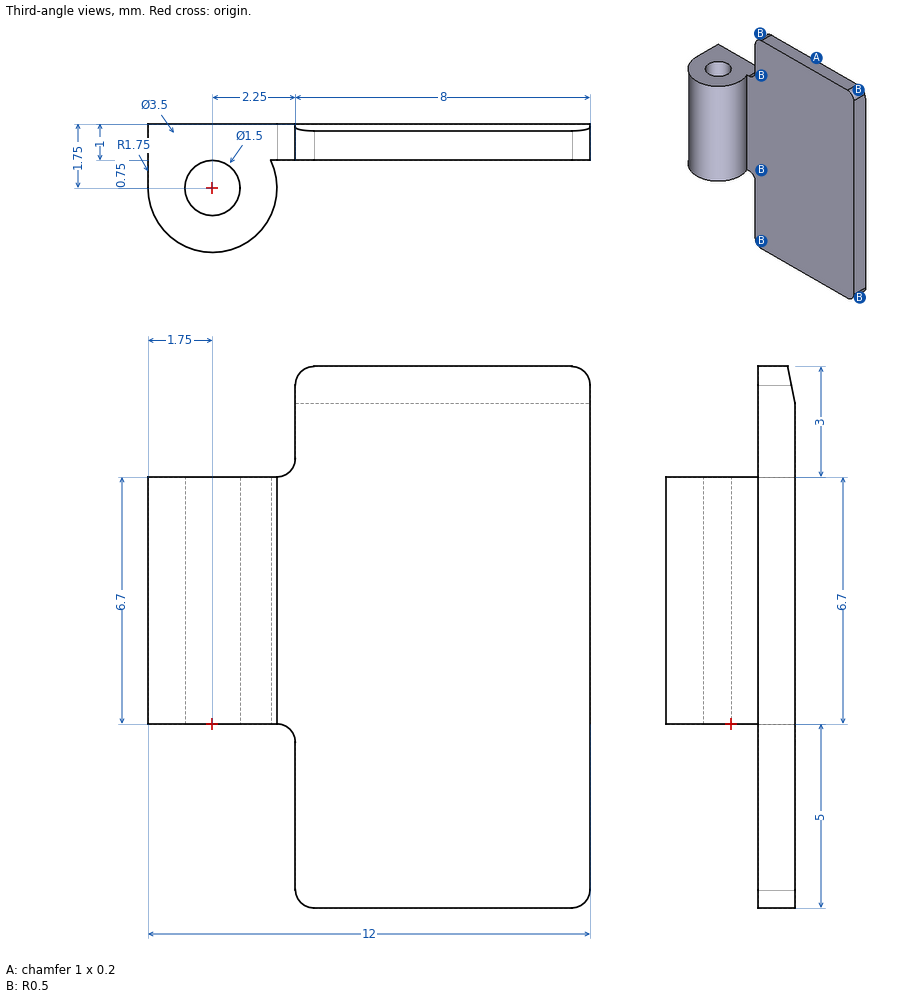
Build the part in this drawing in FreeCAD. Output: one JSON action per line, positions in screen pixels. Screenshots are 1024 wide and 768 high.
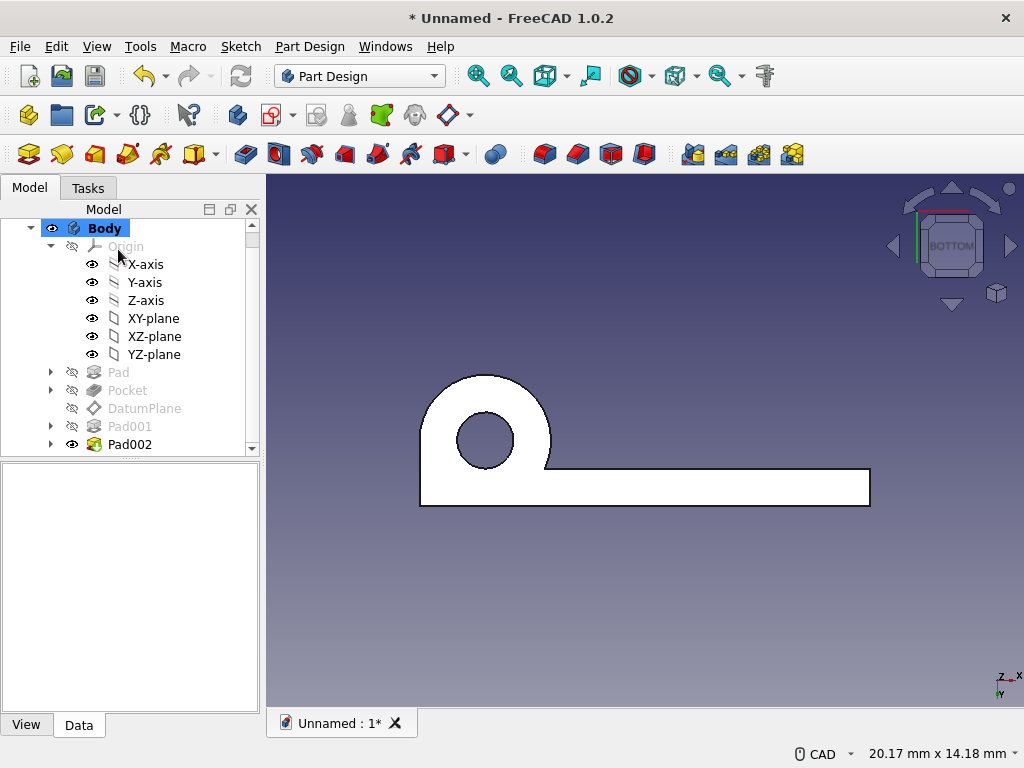
{"action": "key", "text": "0"}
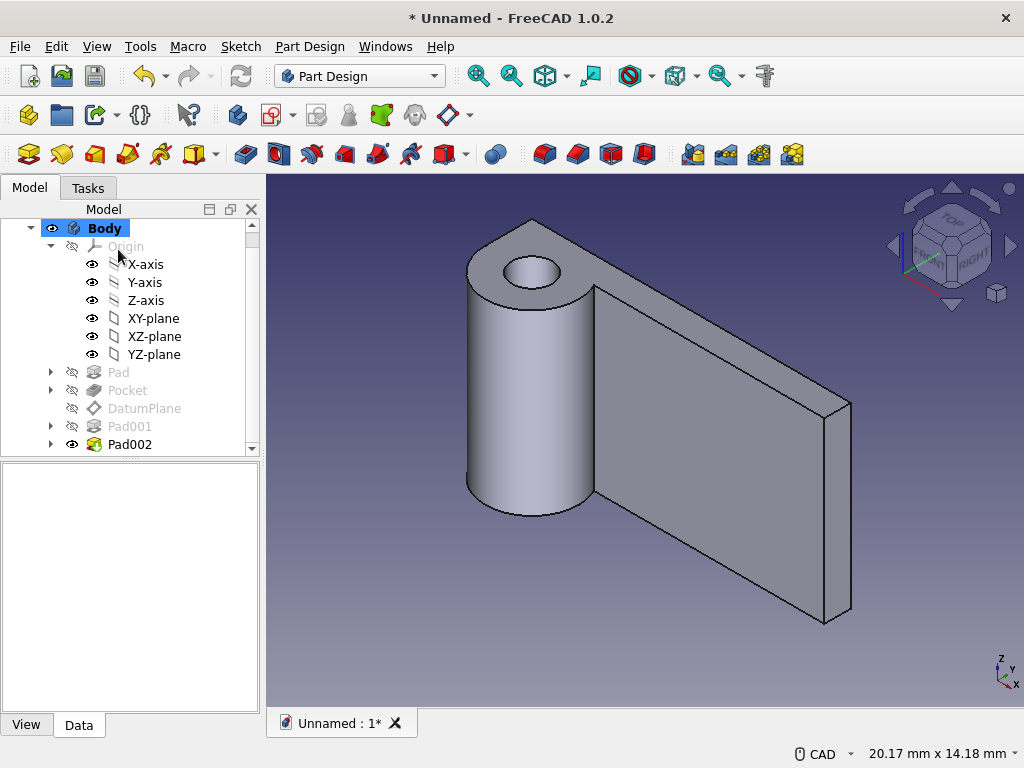
{"action": "left_click", "coordinate": [535, 242]}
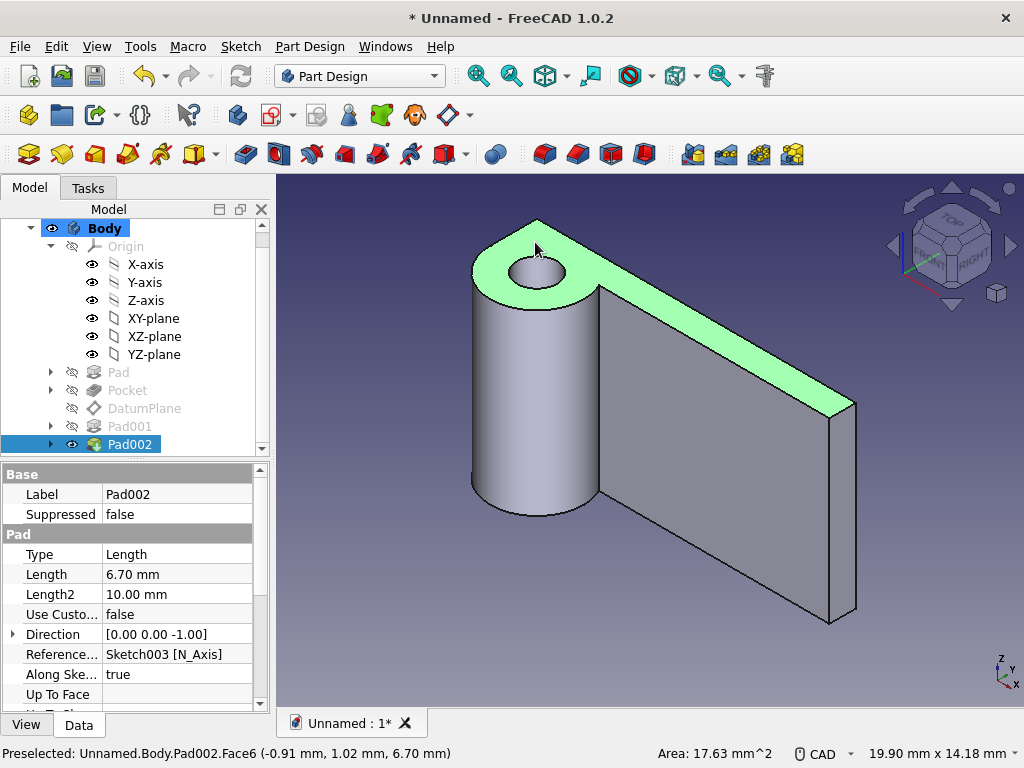
{"action": "left_click", "coordinate": [270, 116]}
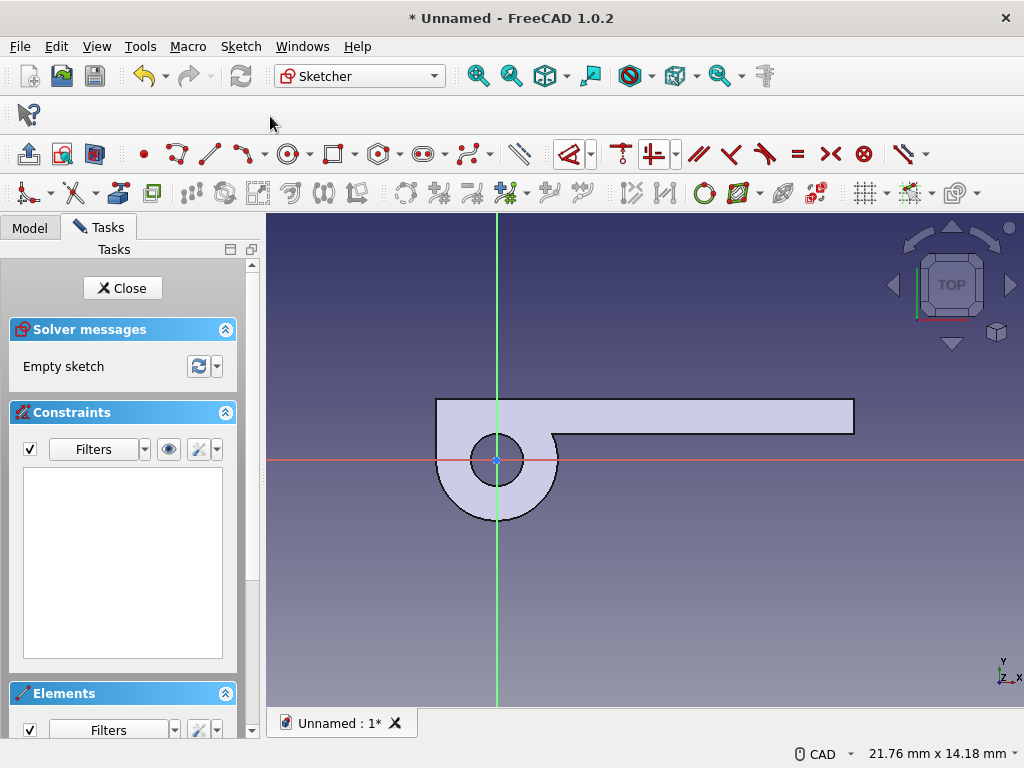
{"action": "scroll", "coordinate": [294, 598], "scroll_direction": "down", "scroll_amount": 1}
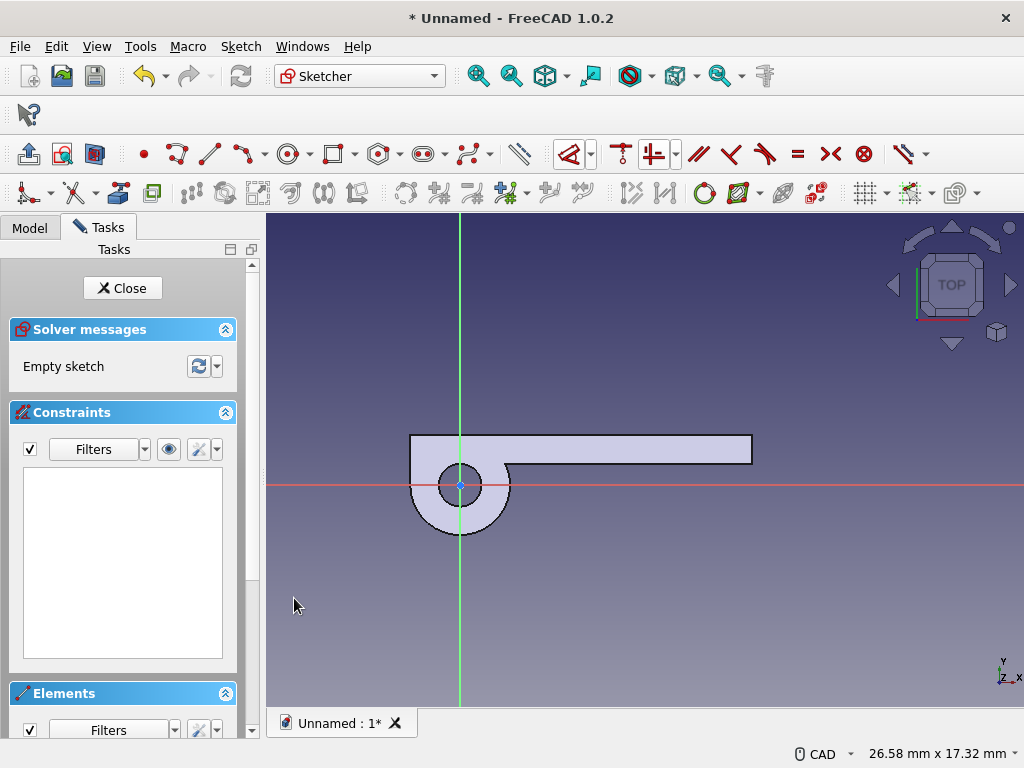
{"action": "scroll", "coordinate": [667, 461], "scroll_direction": "up", "scroll_amount": 2}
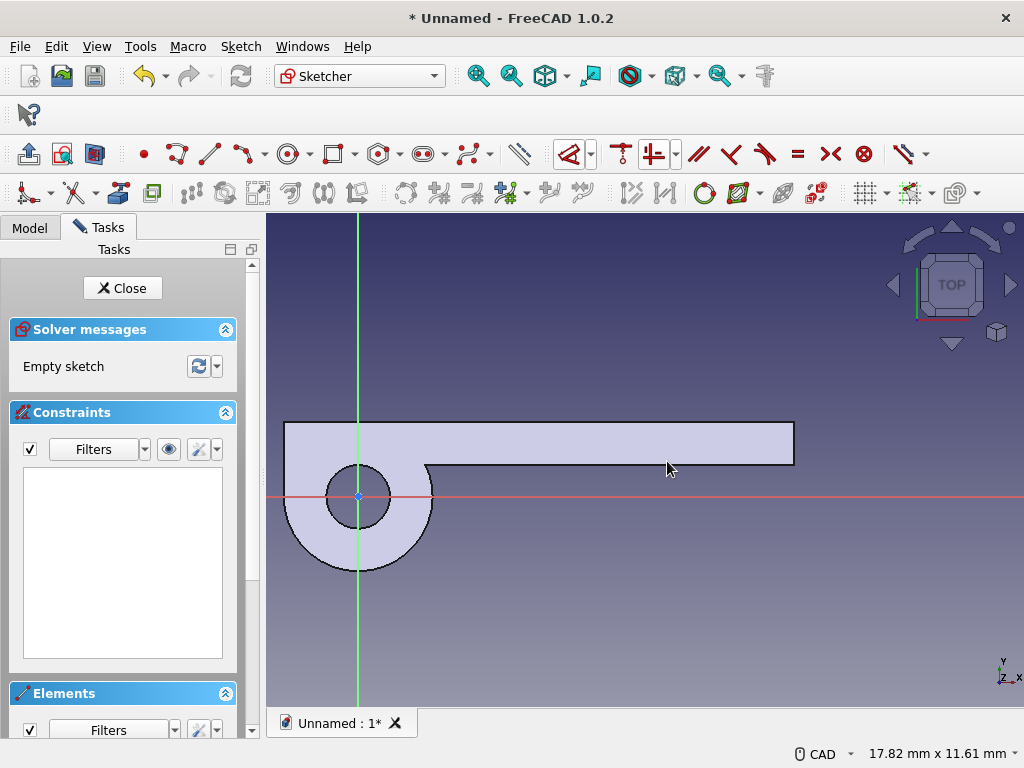
{"action": "left_click", "coordinate": [332, 154]}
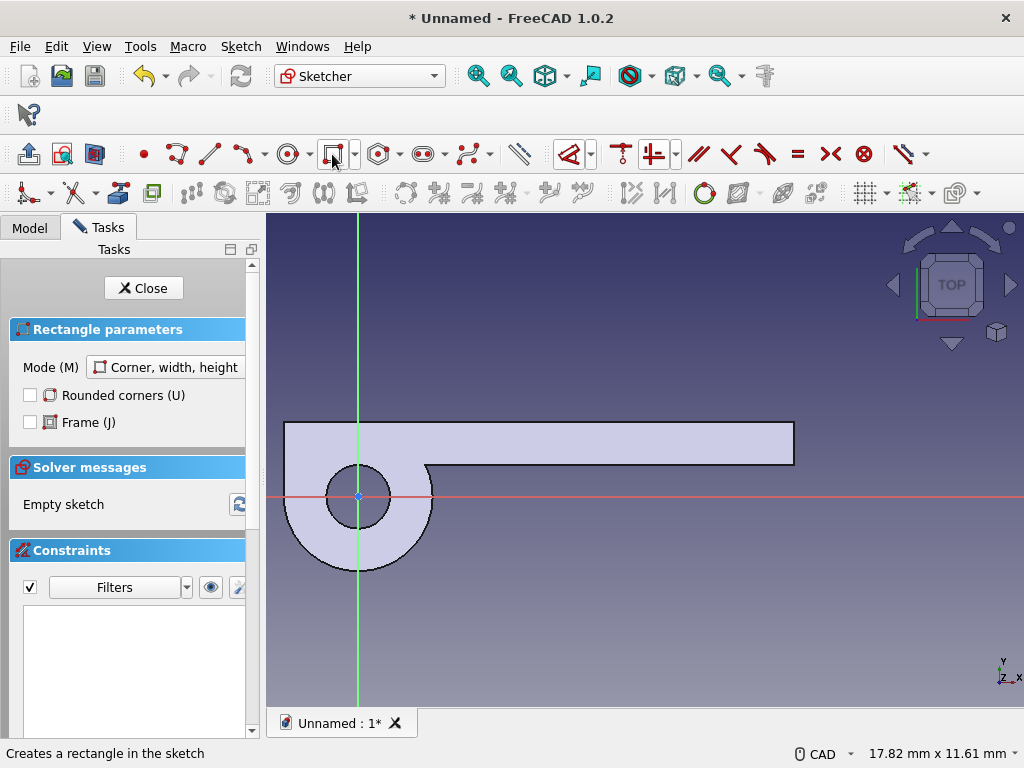
{"action": "left_click", "coordinate": [454, 422]}
{"action": "left_click", "coordinate": [794, 465]}
{"action": "key", "text": "Escape"}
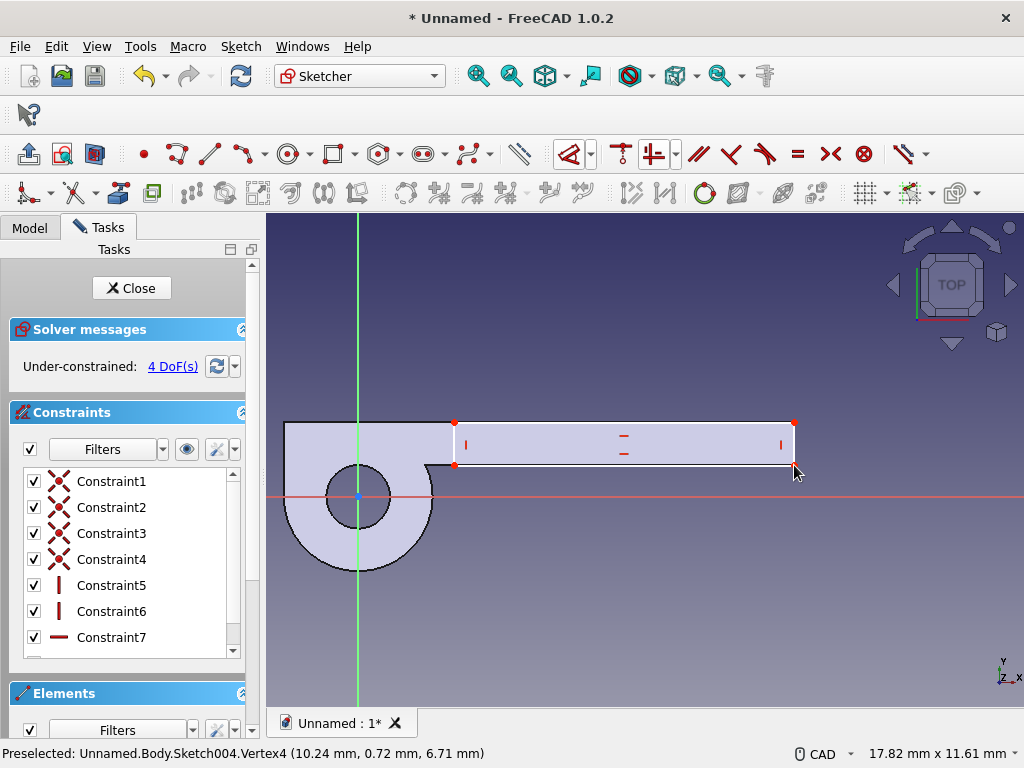
{"action": "left_click", "coordinate": [454, 436]}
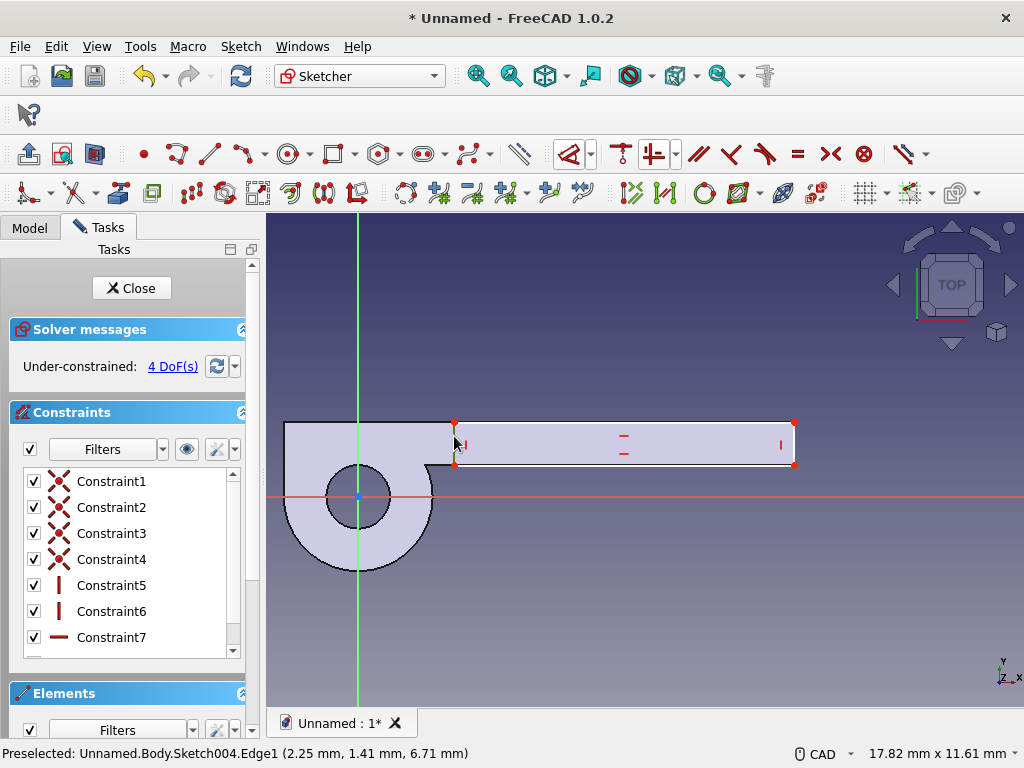
{"action": "left_click", "coordinate": [590, 154]}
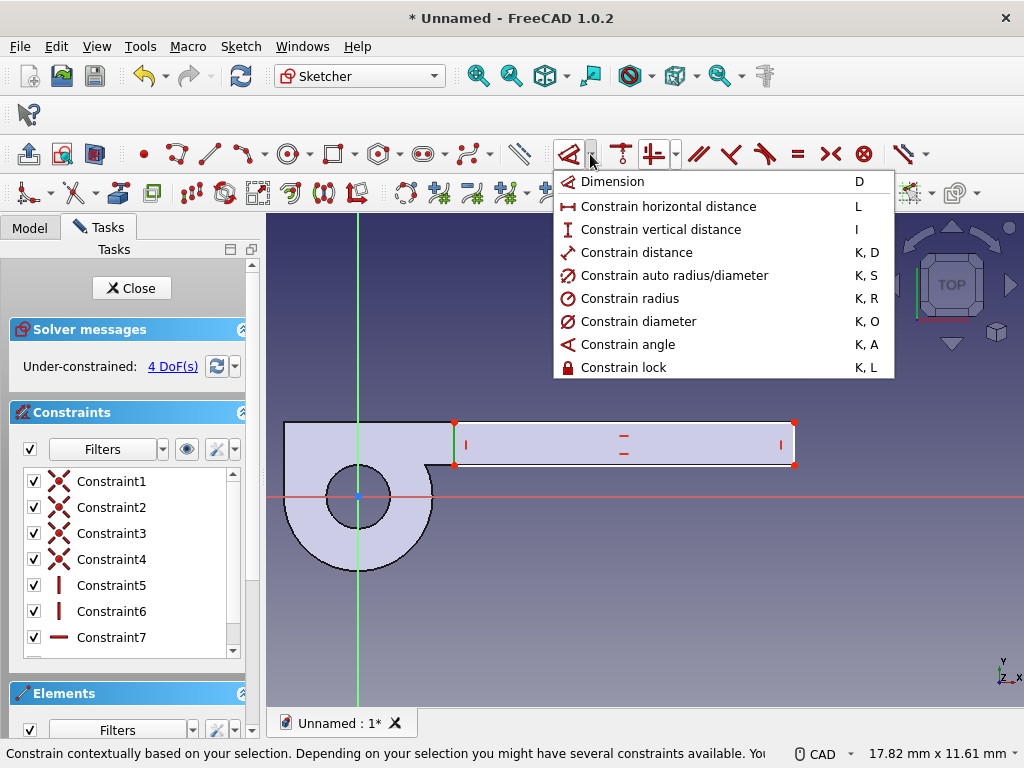
{"action": "left_click", "coordinate": [724, 230]}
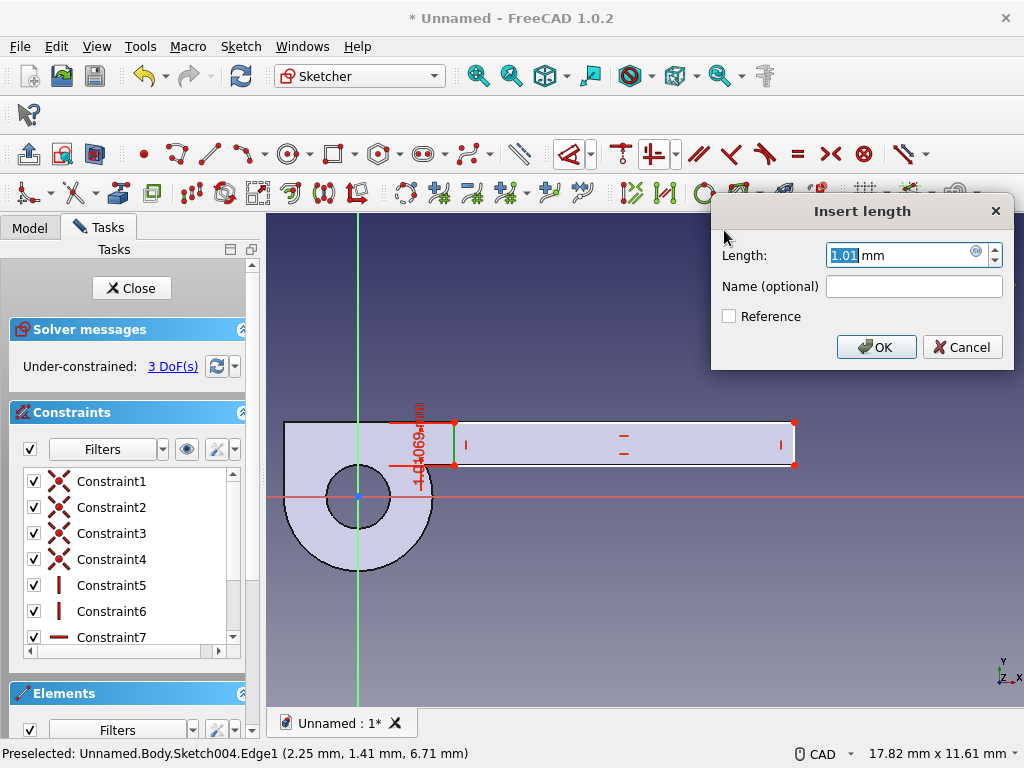
{"action": "type", "text": "1"}
{"action": "key", "text": "Return"}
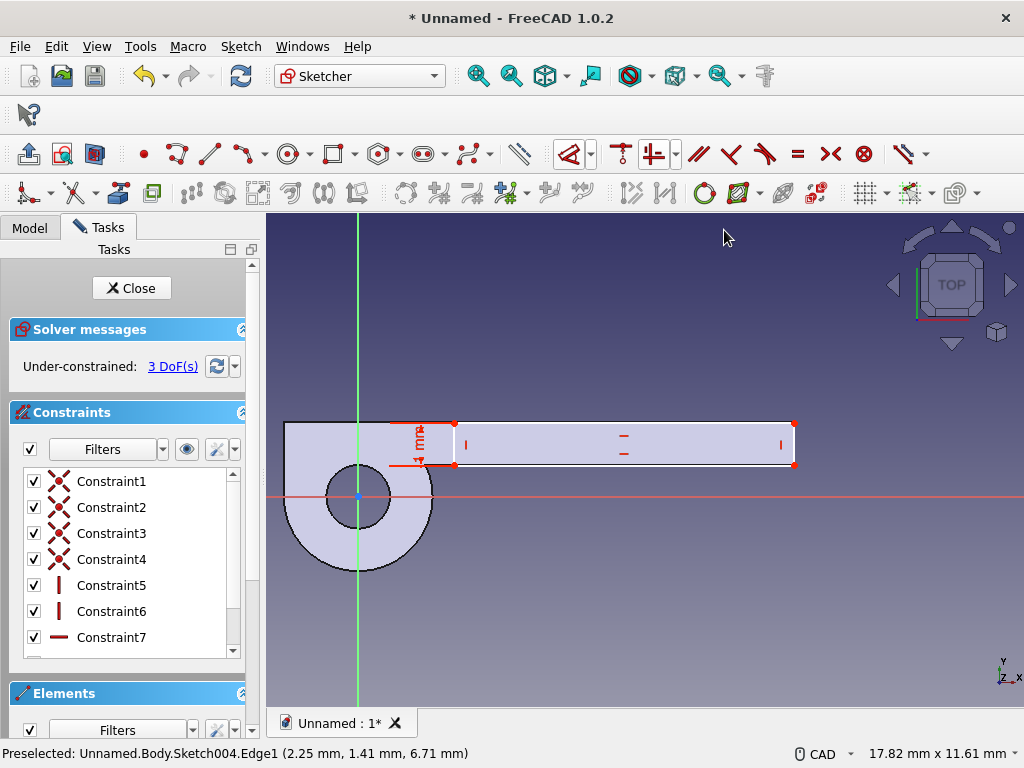
{"action": "left_click", "coordinate": [556, 466]}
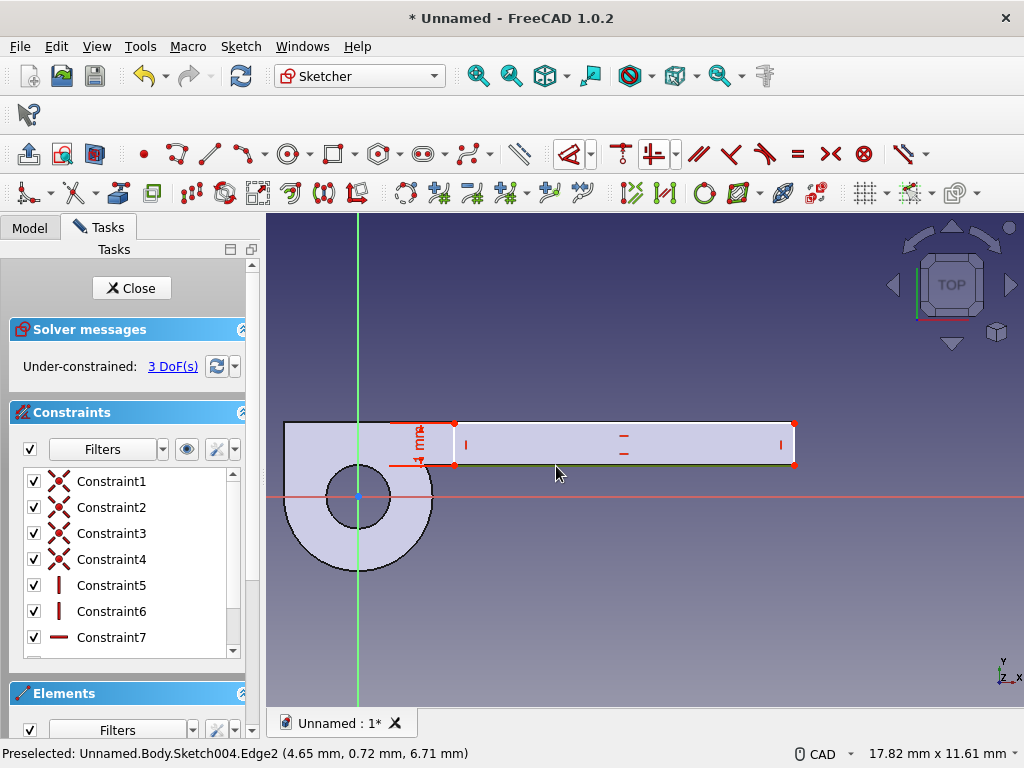
{"action": "left_click", "coordinate": [590, 154]}